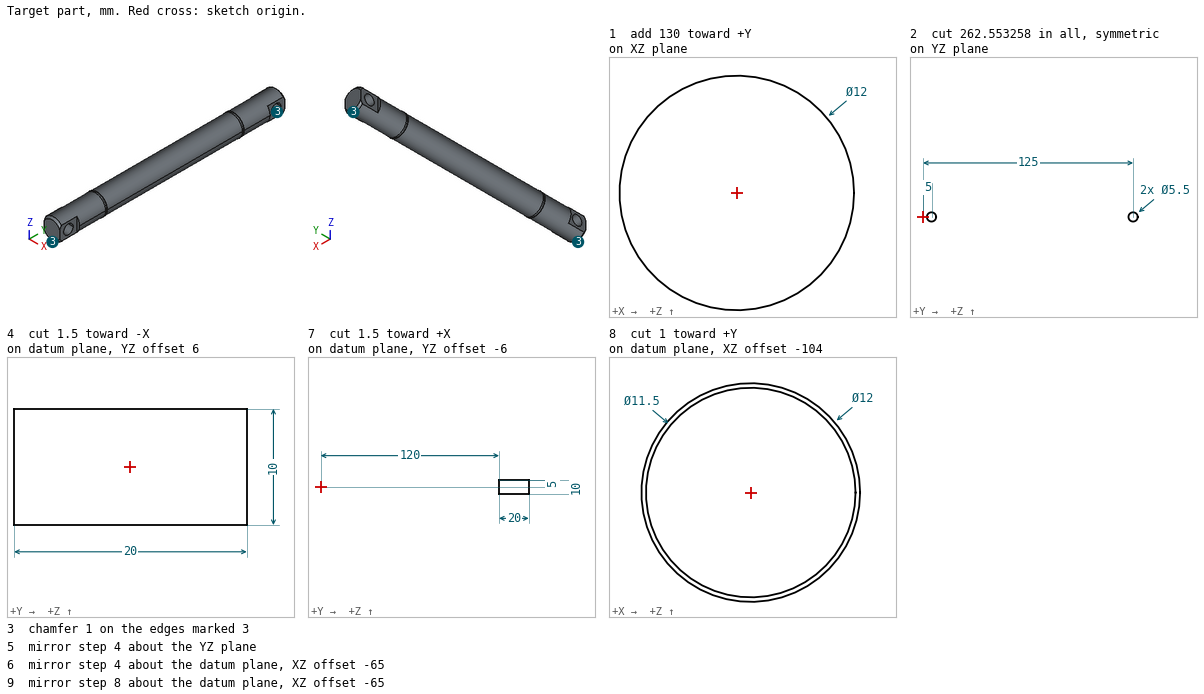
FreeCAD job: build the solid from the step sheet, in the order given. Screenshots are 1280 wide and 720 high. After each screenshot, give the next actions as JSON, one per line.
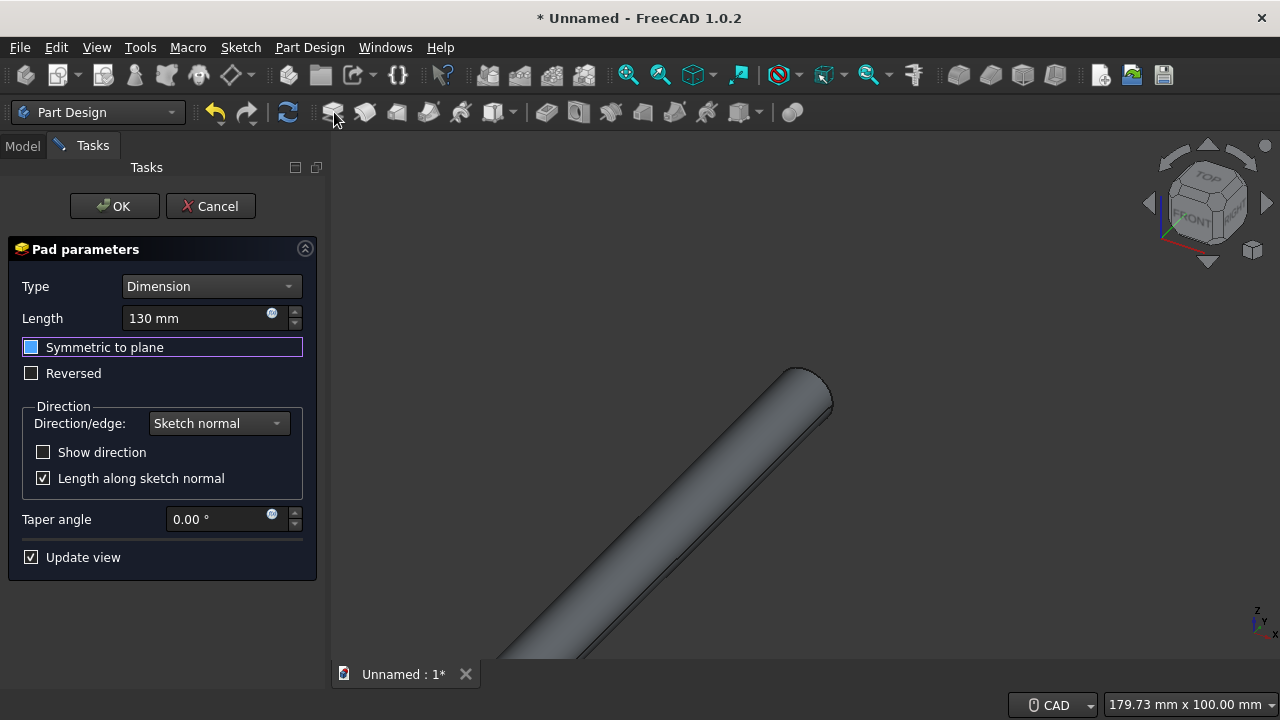
{"action": "left_click", "coordinate": [30, 373]}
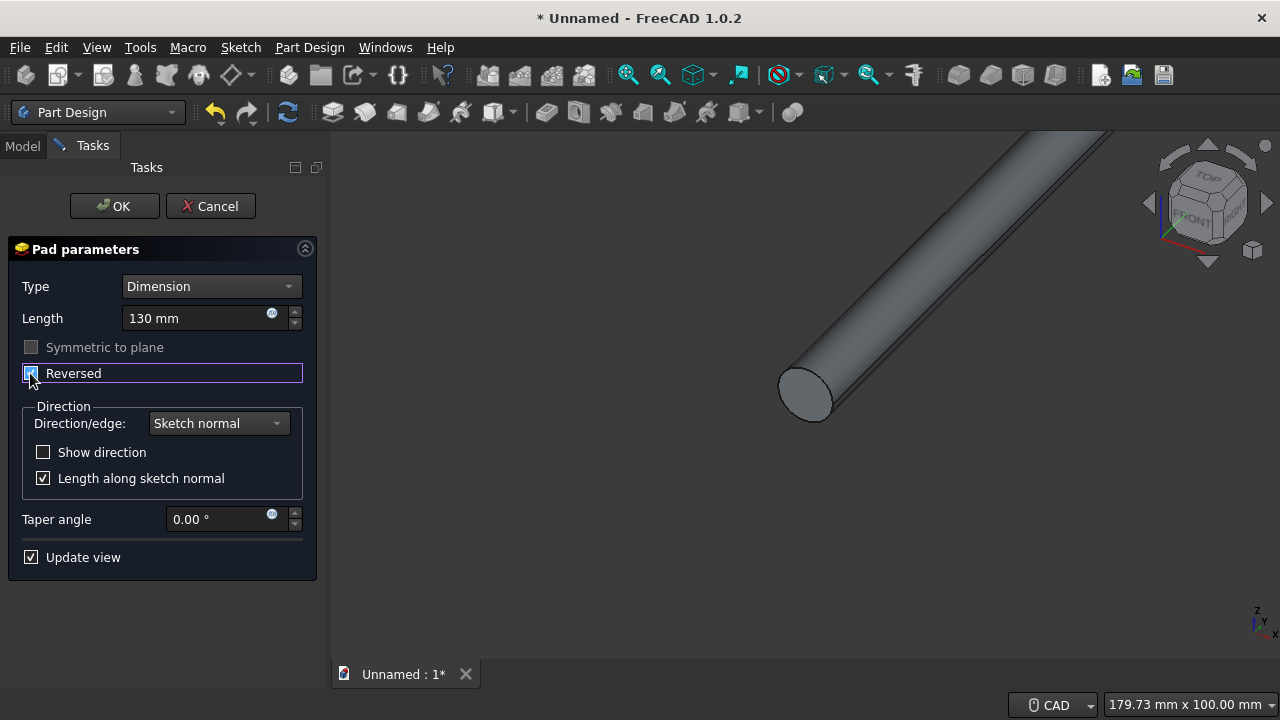
{"action": "left_click", "coordinate": [115, 206]}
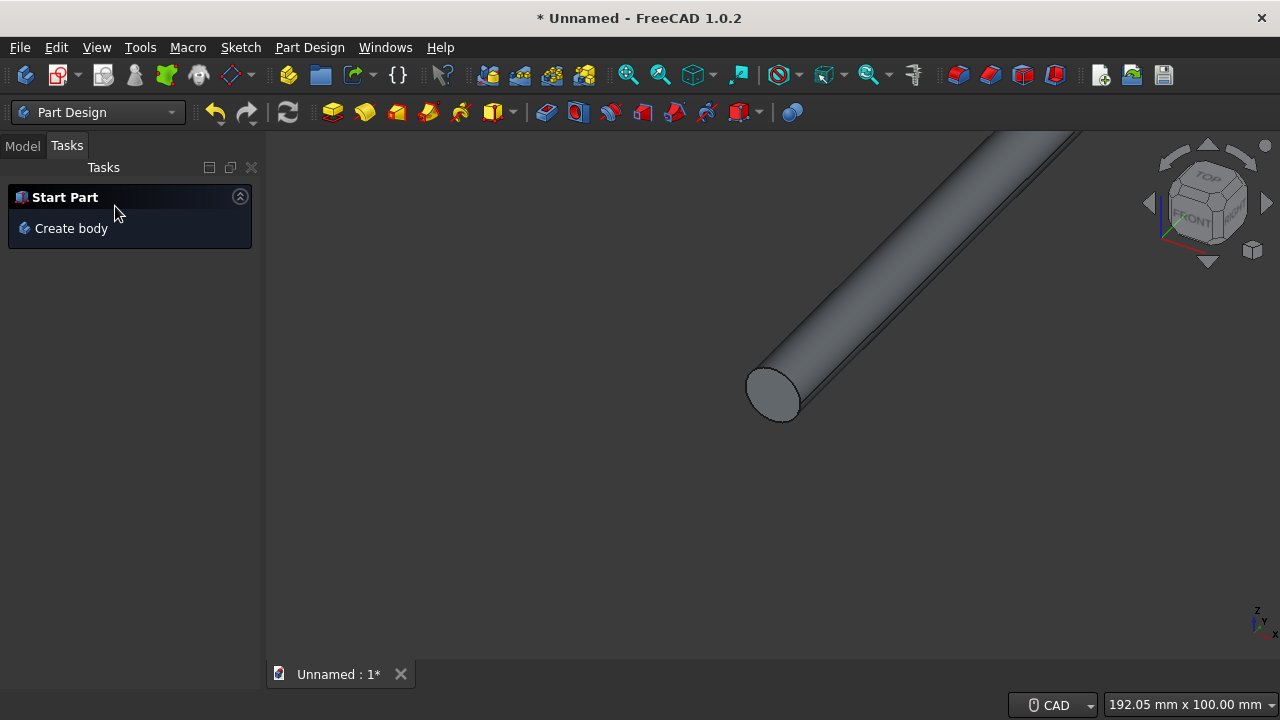
{"action": "key", "text": "v f"}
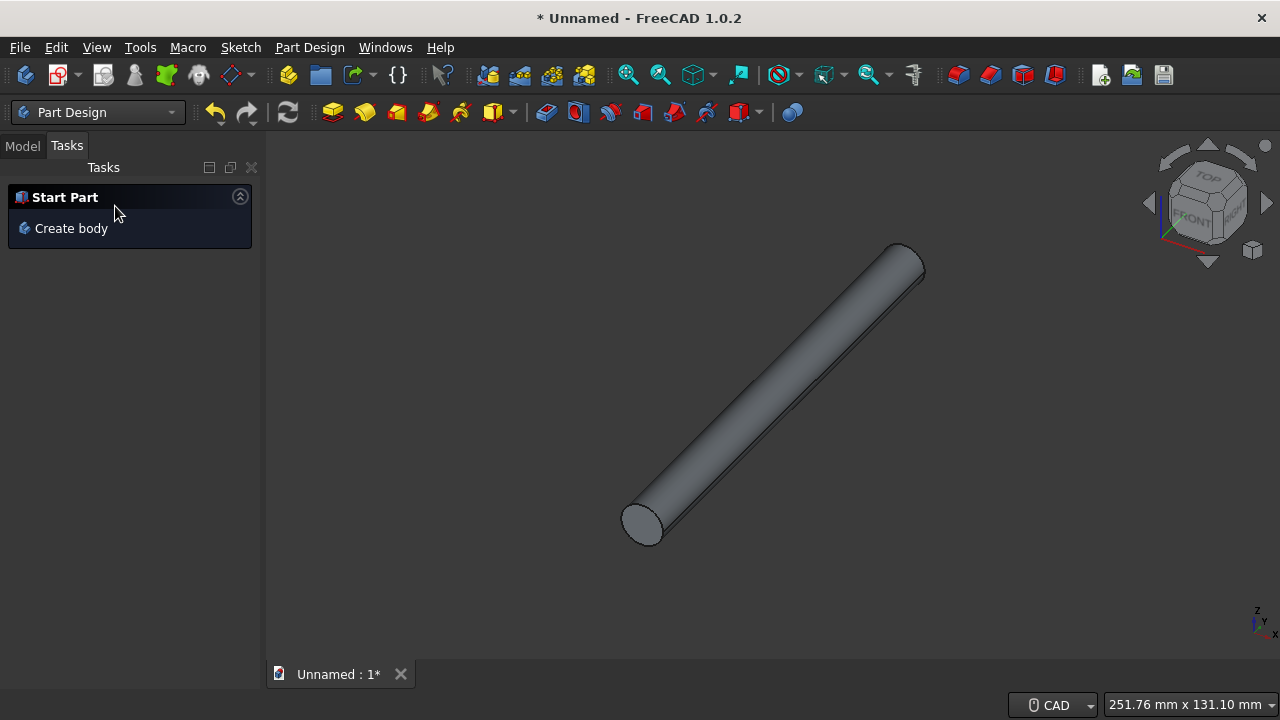
{"action": "left_click", "coordinate": [58, 76]}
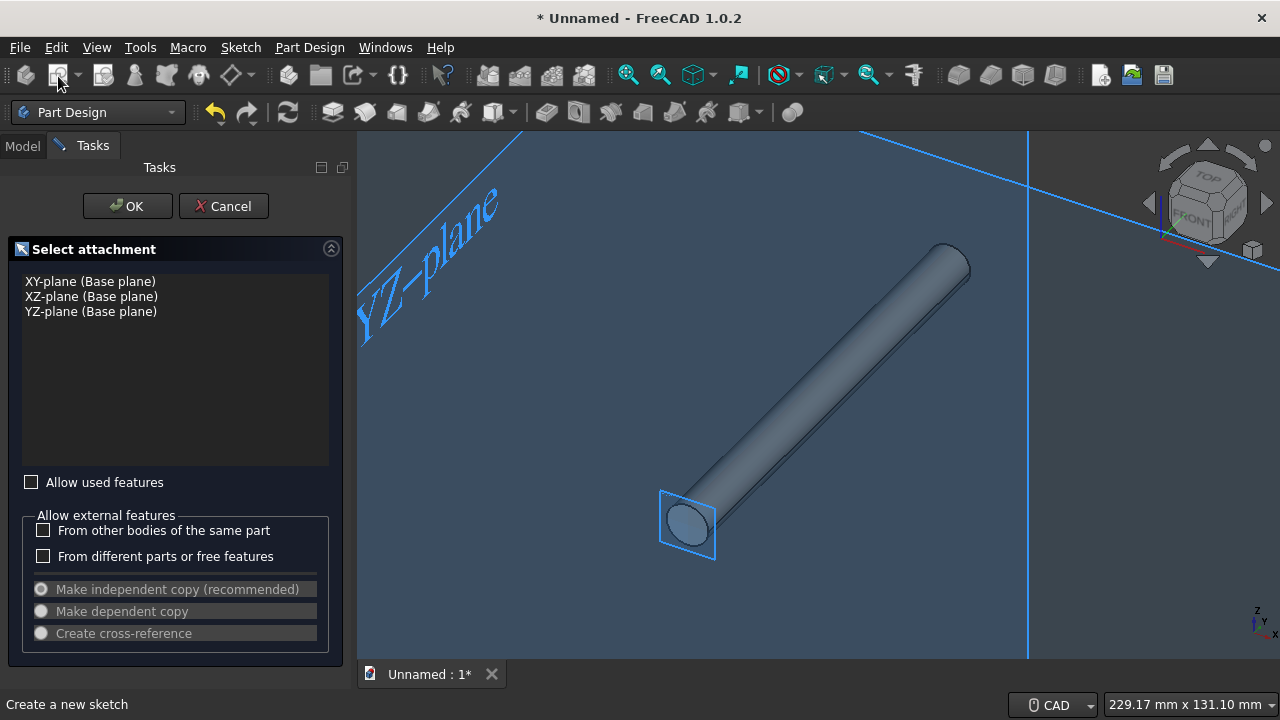
{"action": "left_click", "coordinate": [82, 312]}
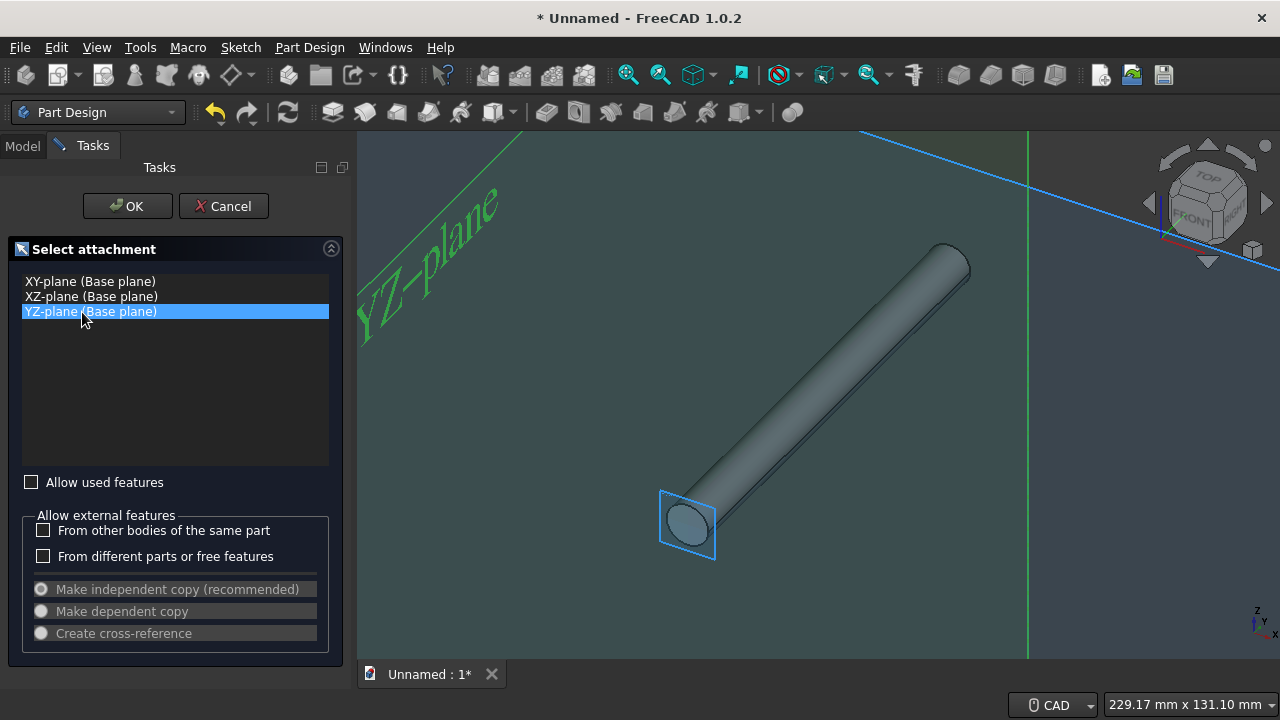
{"action": "left_click", "coordinate": [128, 206]}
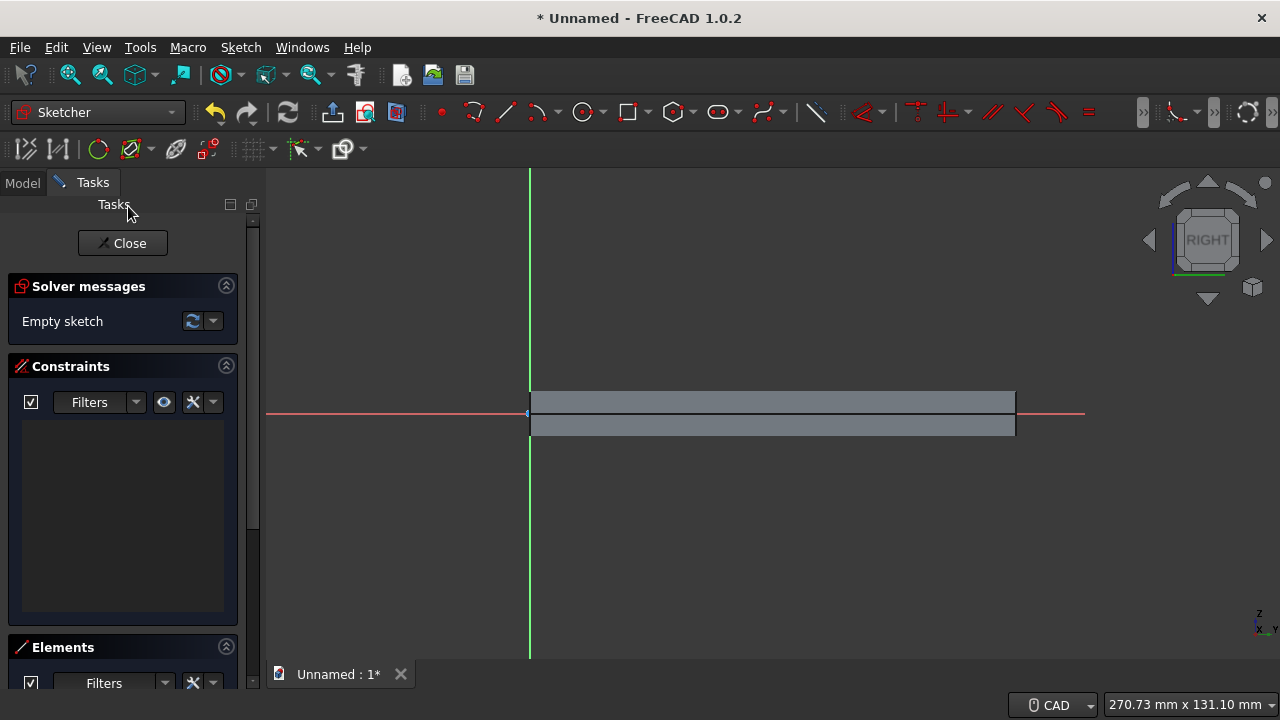
{"action": "key", "text": "q s"}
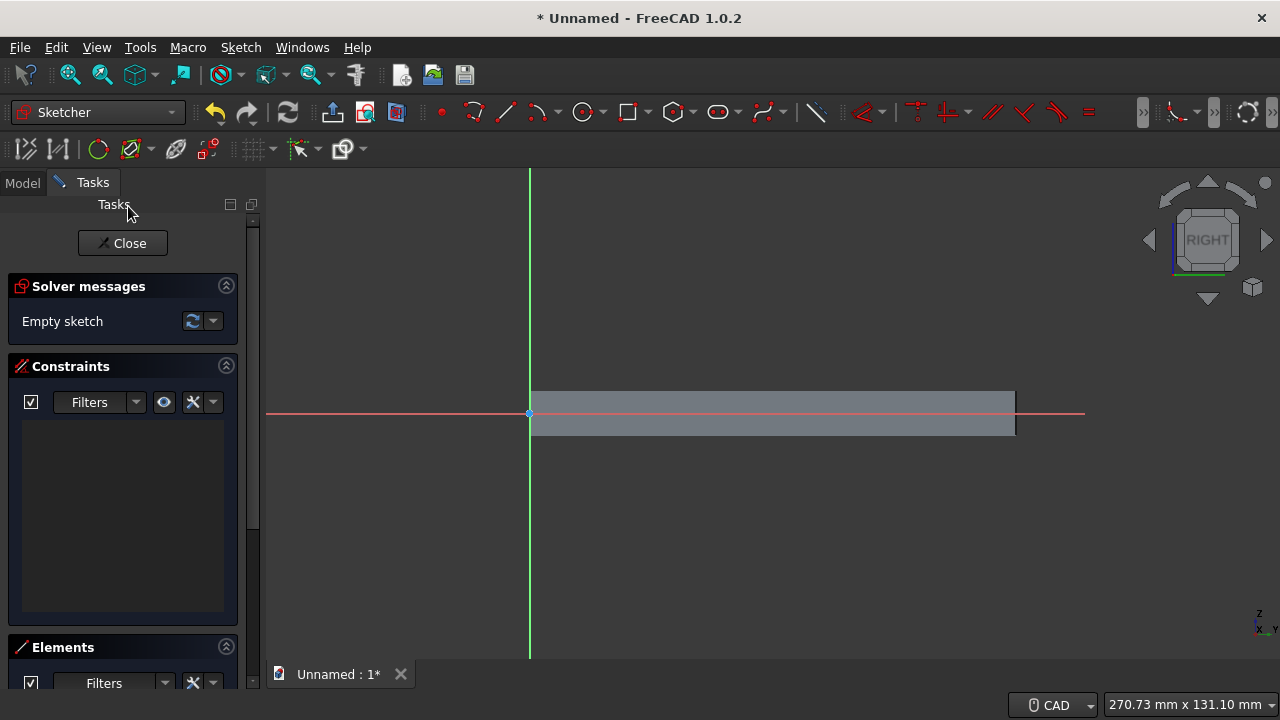
{"action": "key", "text": "g c"}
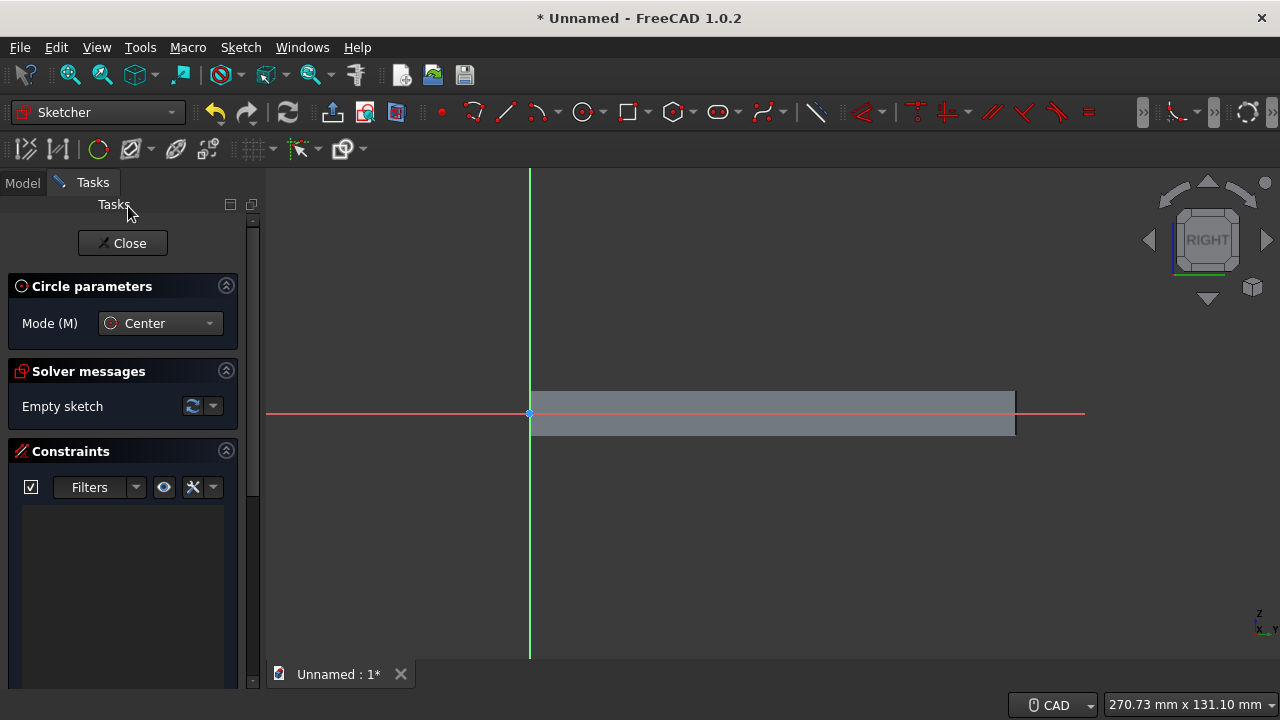
{"action": "scroll", "coordinate": [998, 414], "scroll_direction": "up", "scroll_amount": 4}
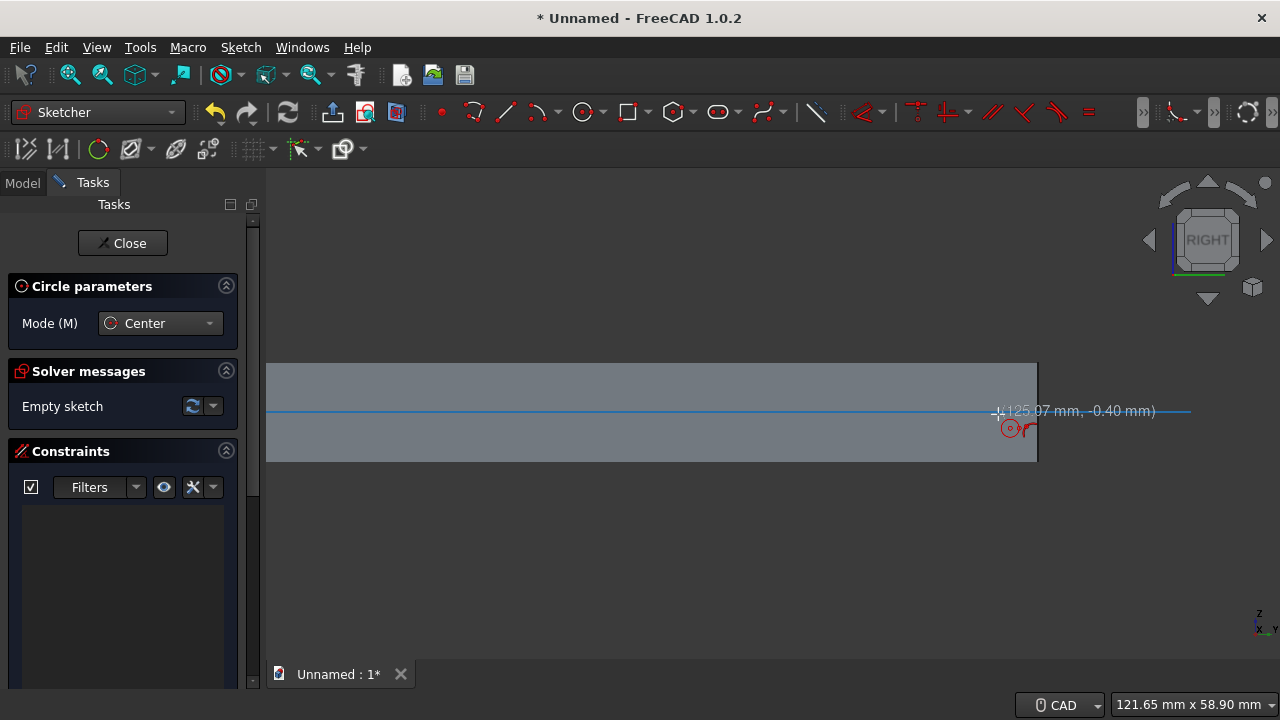
{"action": "left_click", "coordinate": [996, 412]}
{"action": "mouse_move", "coordinate": [1013, 396]}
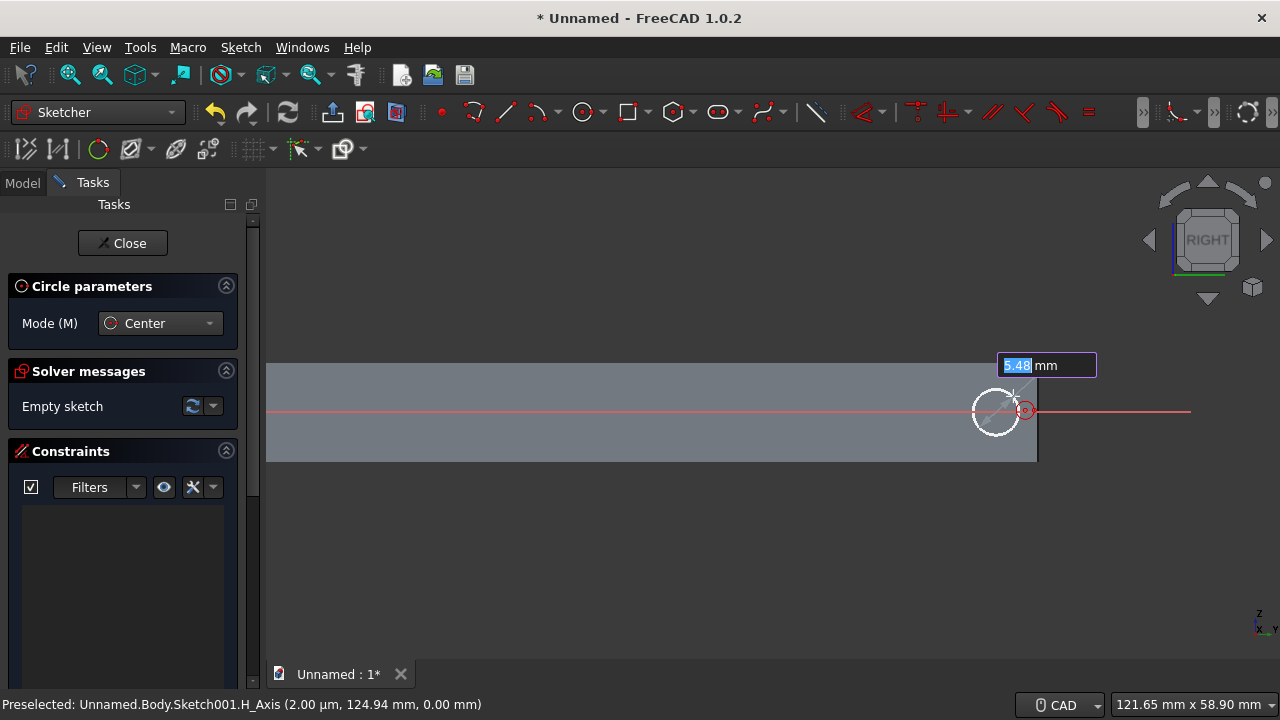
{"action": "type", "text": "5.5"}
{"action": "key", "text": "Return"}